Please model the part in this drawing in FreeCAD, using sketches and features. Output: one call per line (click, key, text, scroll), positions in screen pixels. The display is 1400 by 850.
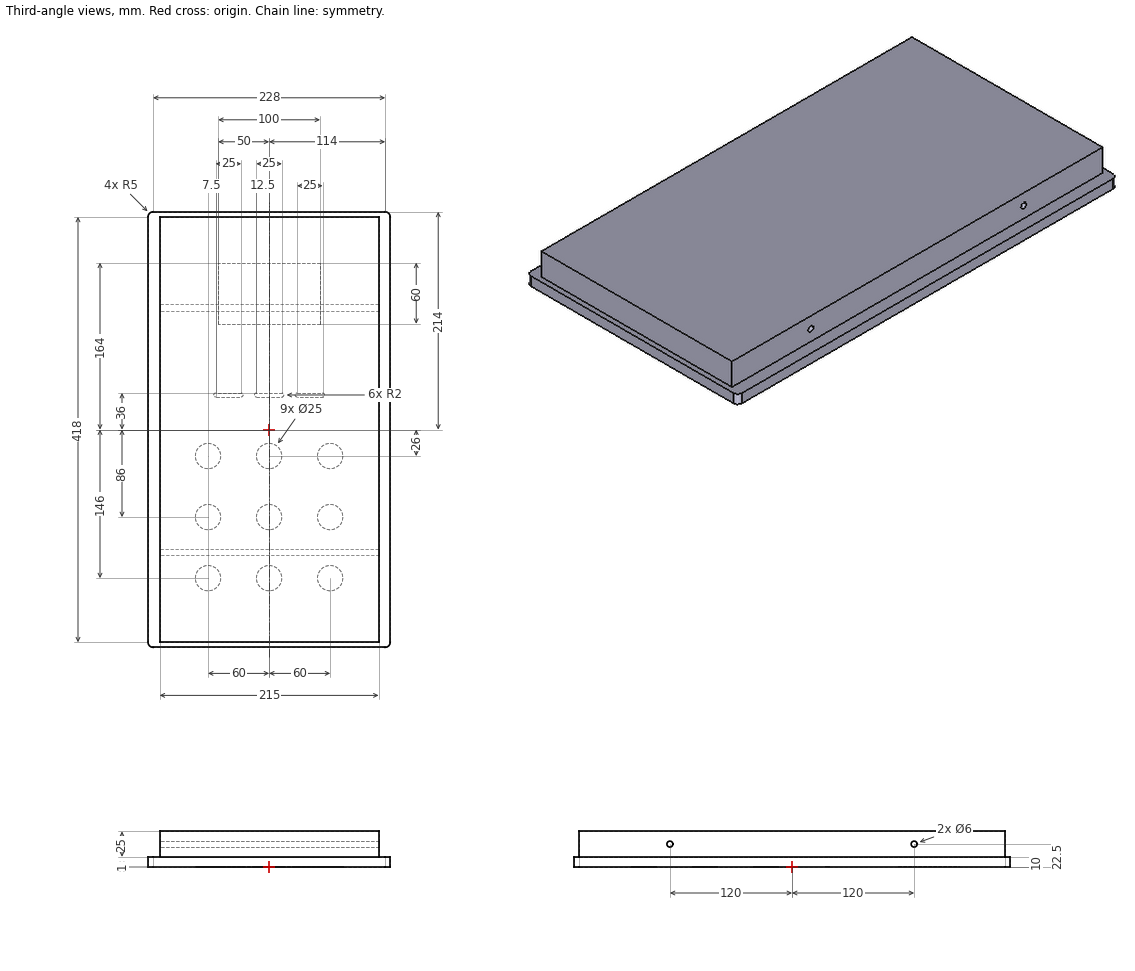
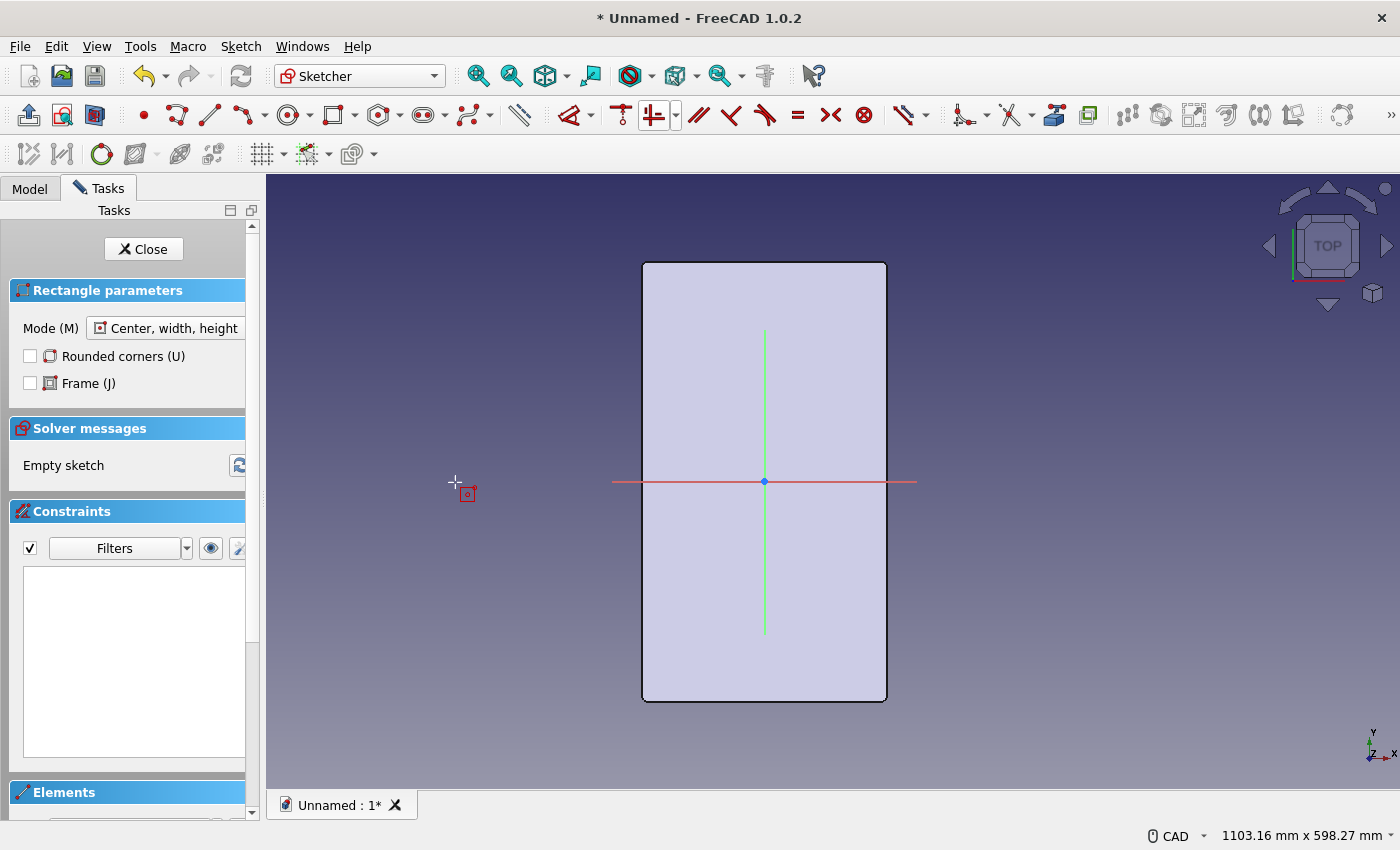
click(765, 482)
move(875, 267)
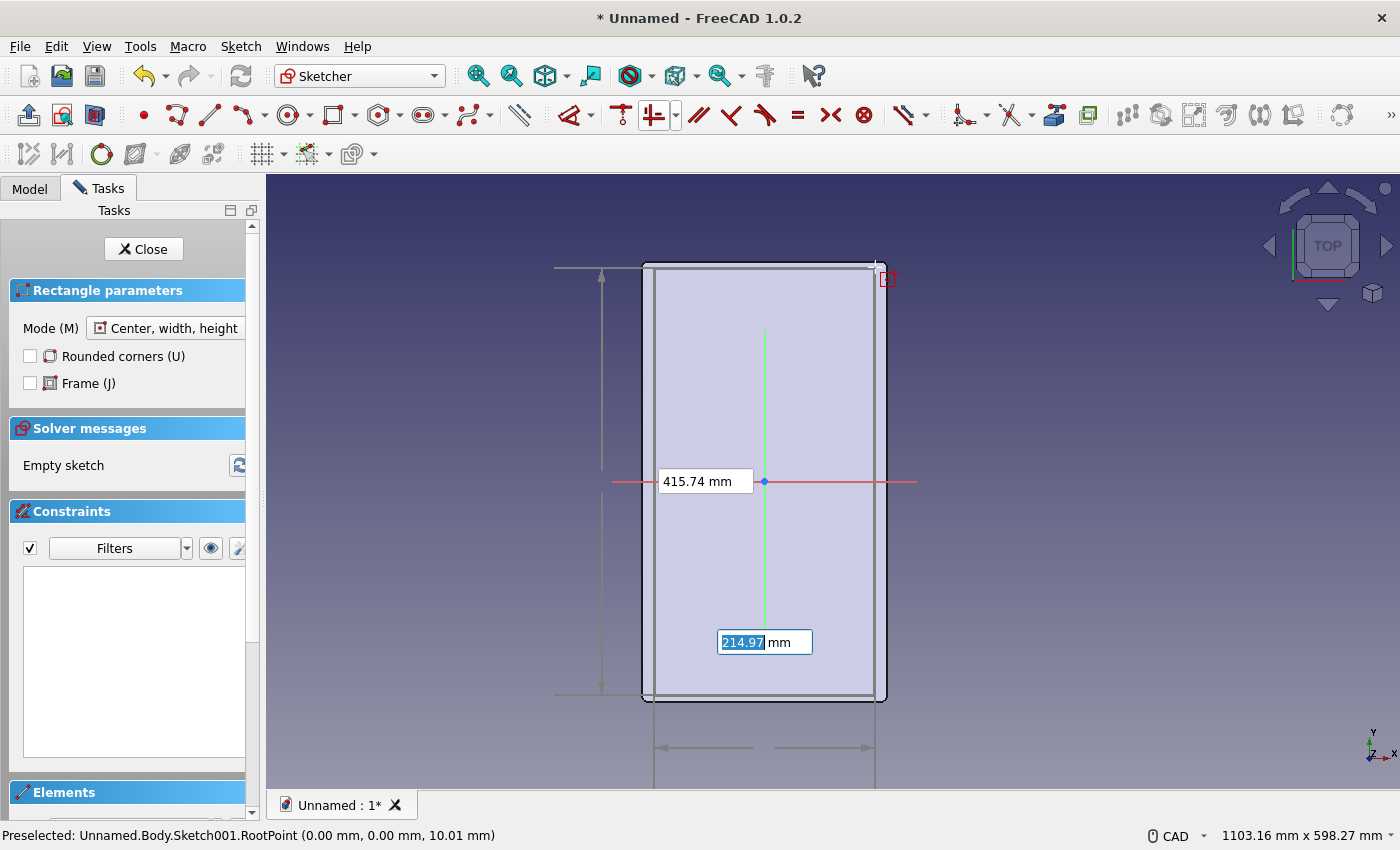
text(215)
key(Tab)
text(418)
key(Return)
key(Escape)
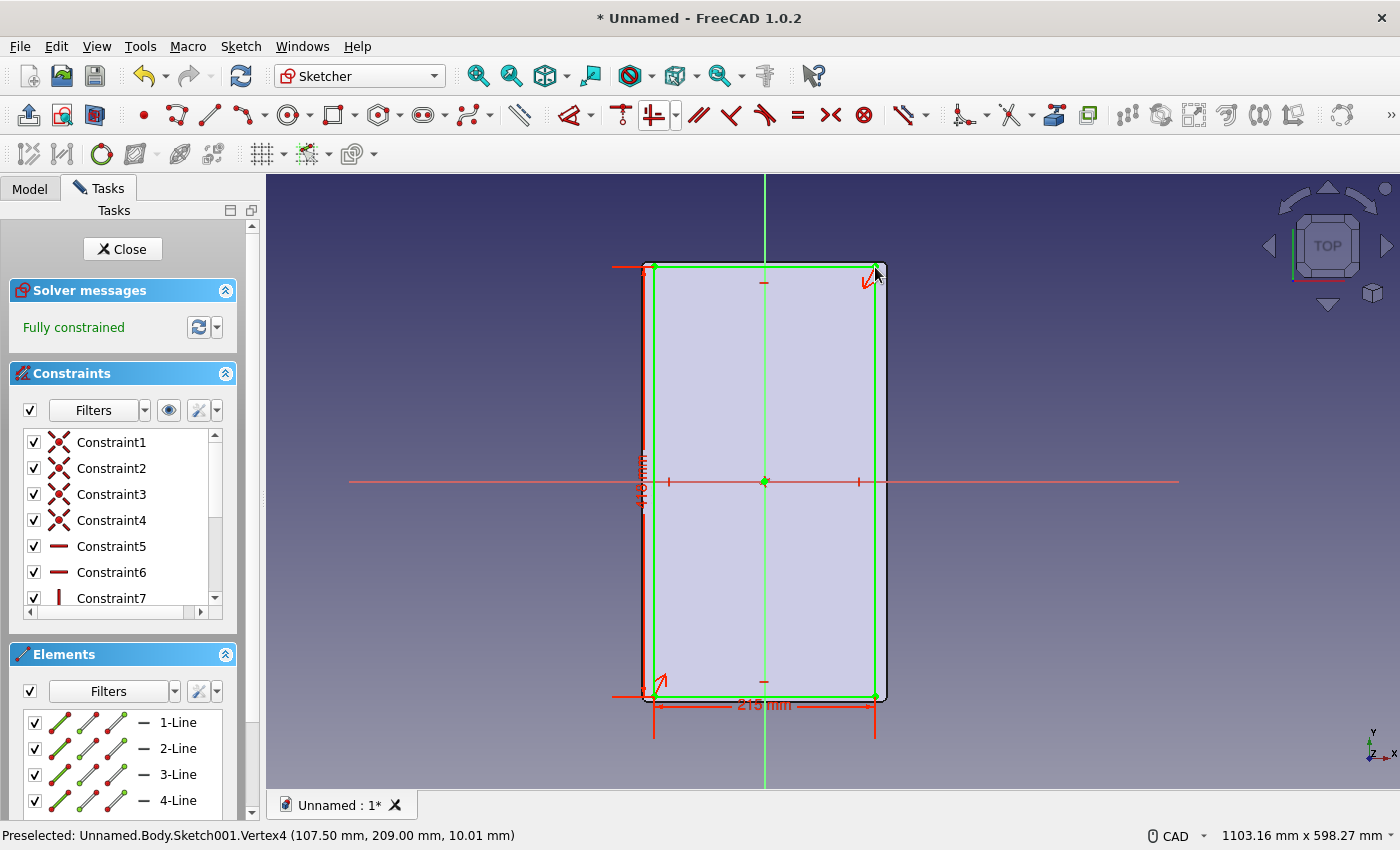
click(123, 249)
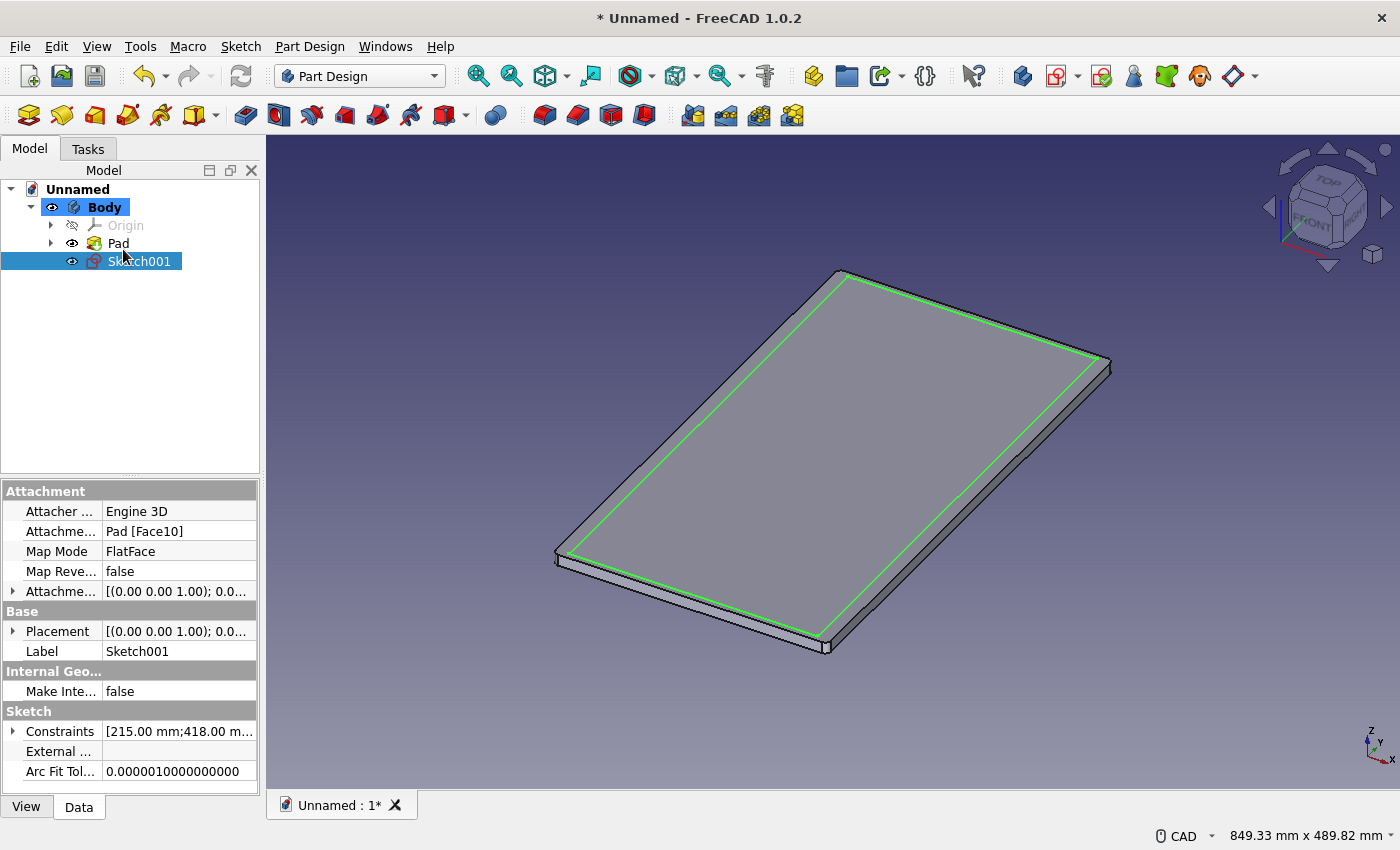
click(29, 116)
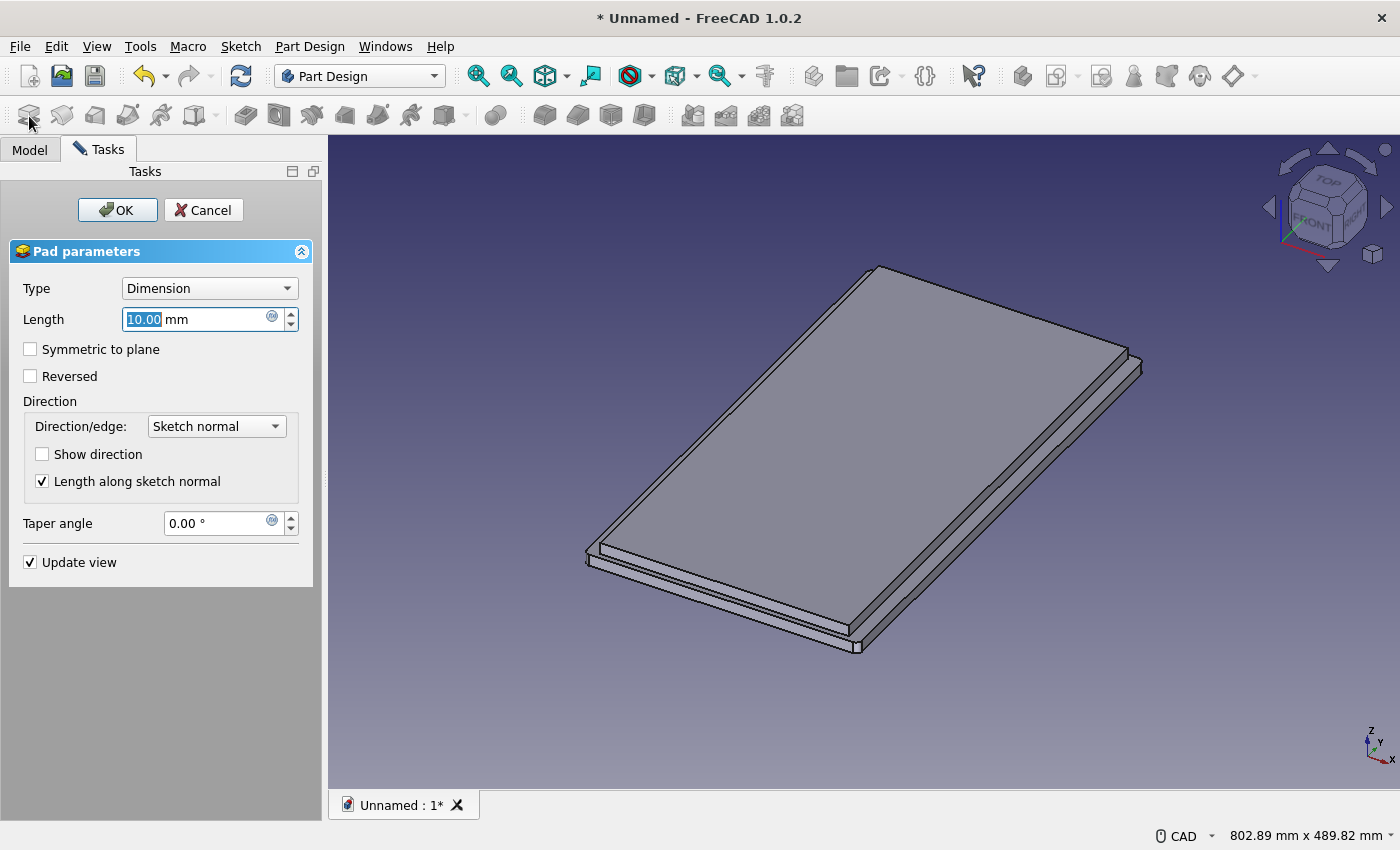
text(25)
key(Tab)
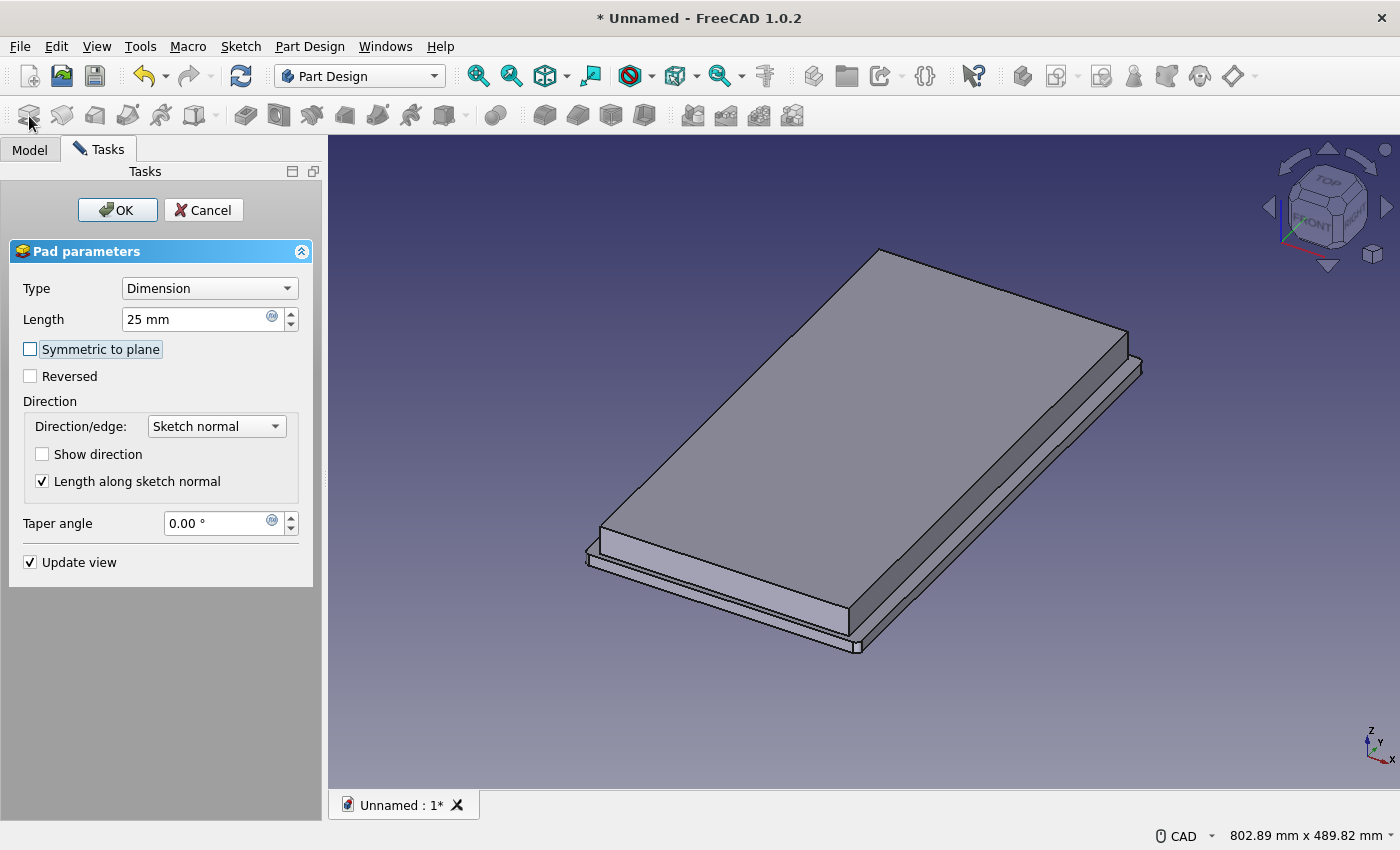
click(118, 210)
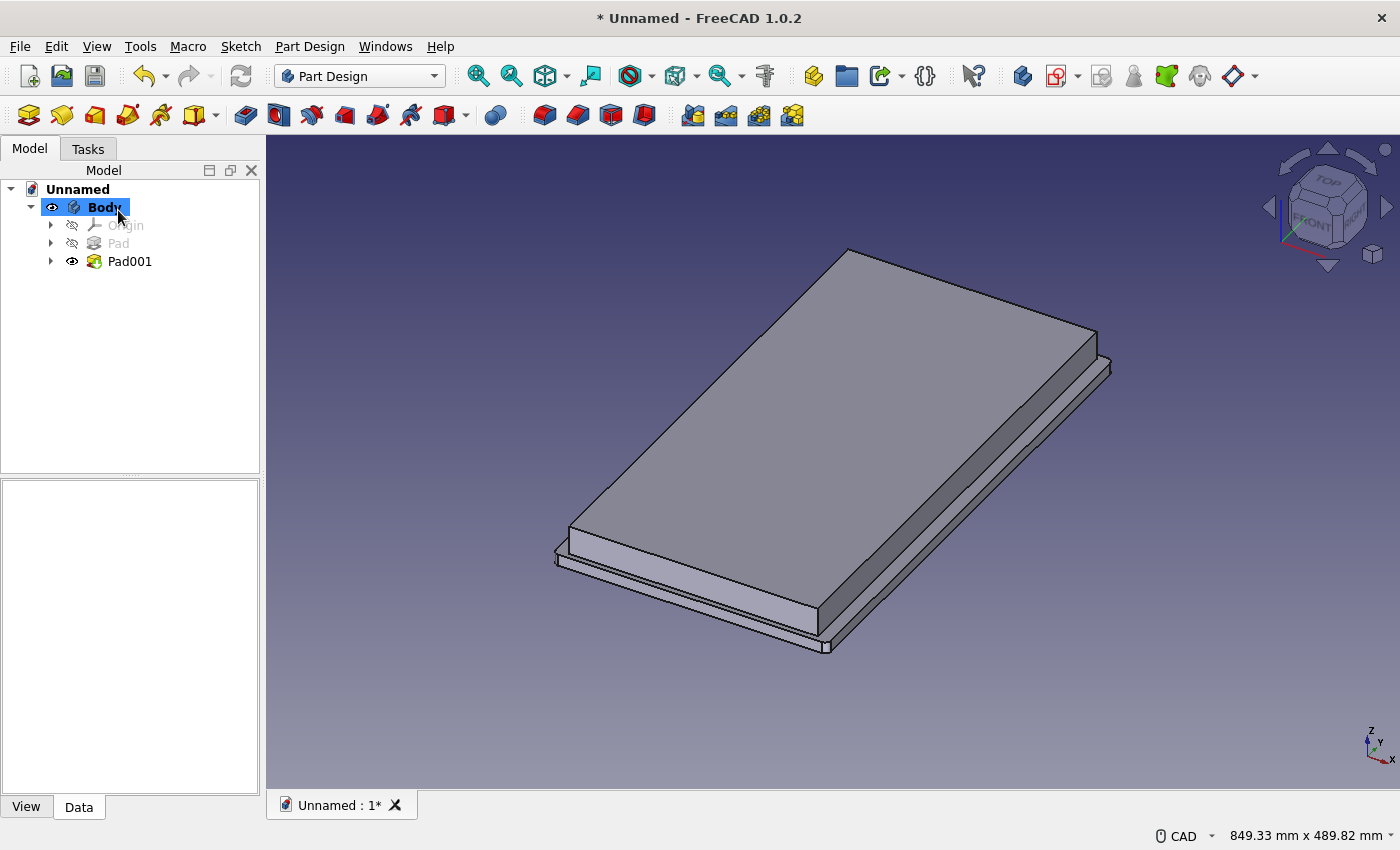
click(1077, 364)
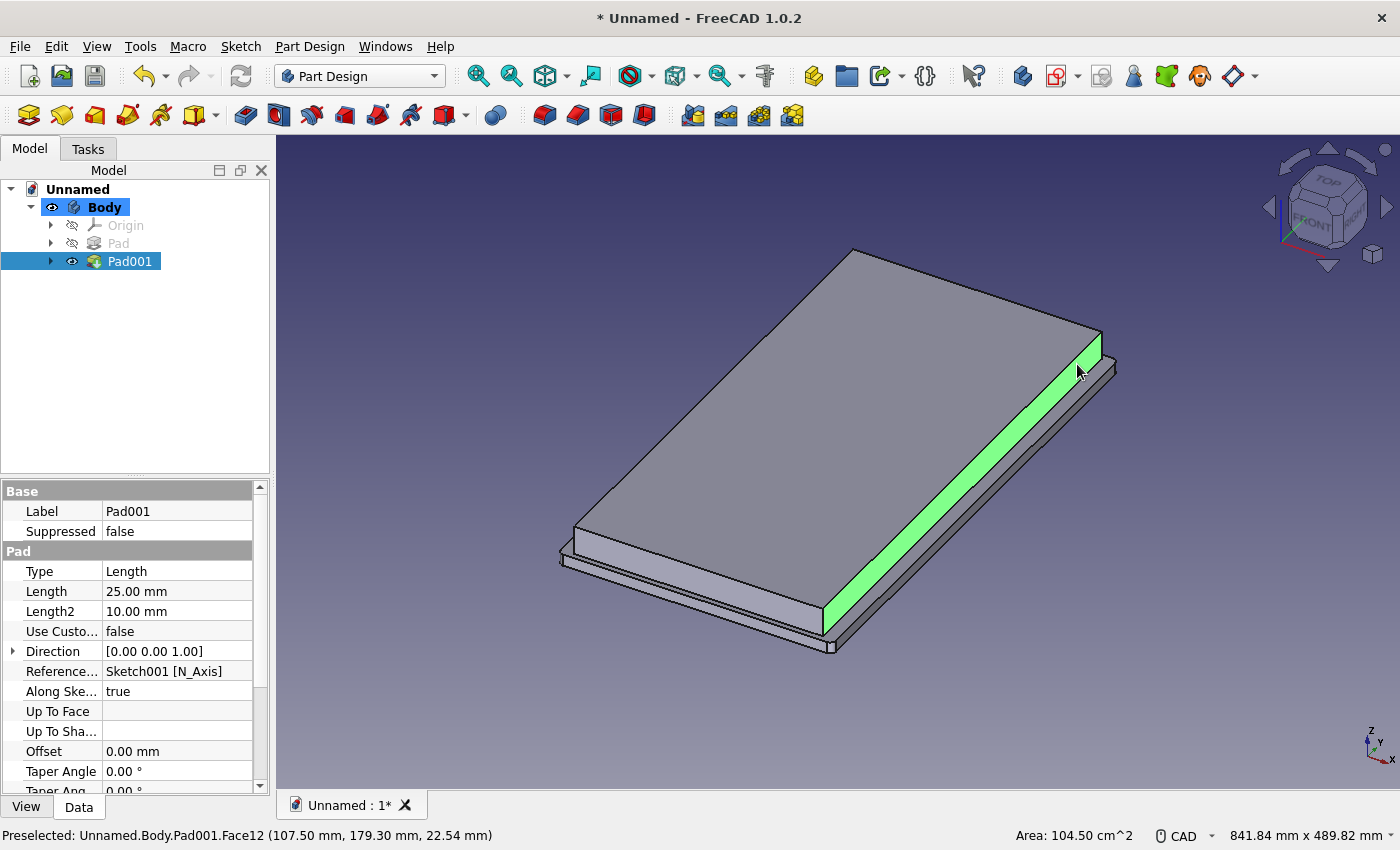
click(1056, 76)